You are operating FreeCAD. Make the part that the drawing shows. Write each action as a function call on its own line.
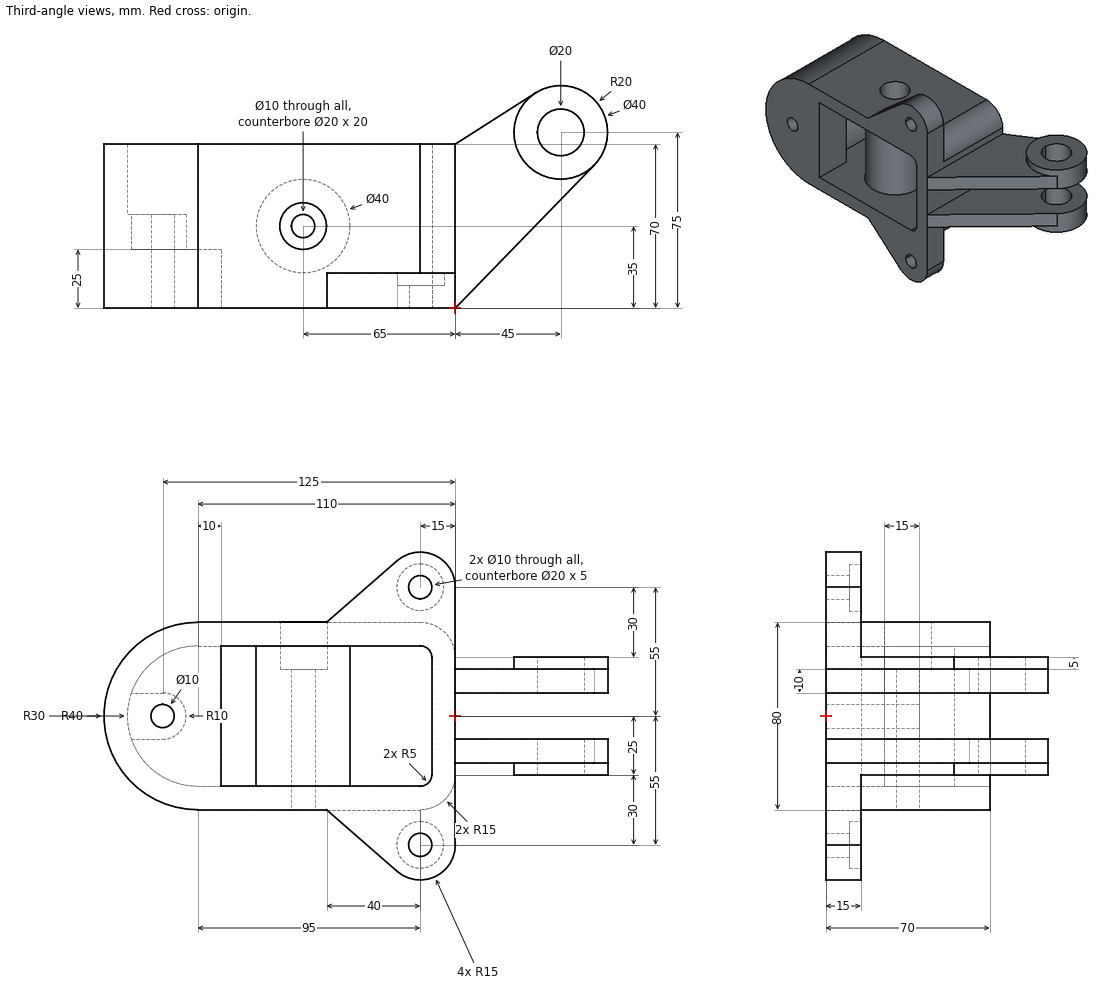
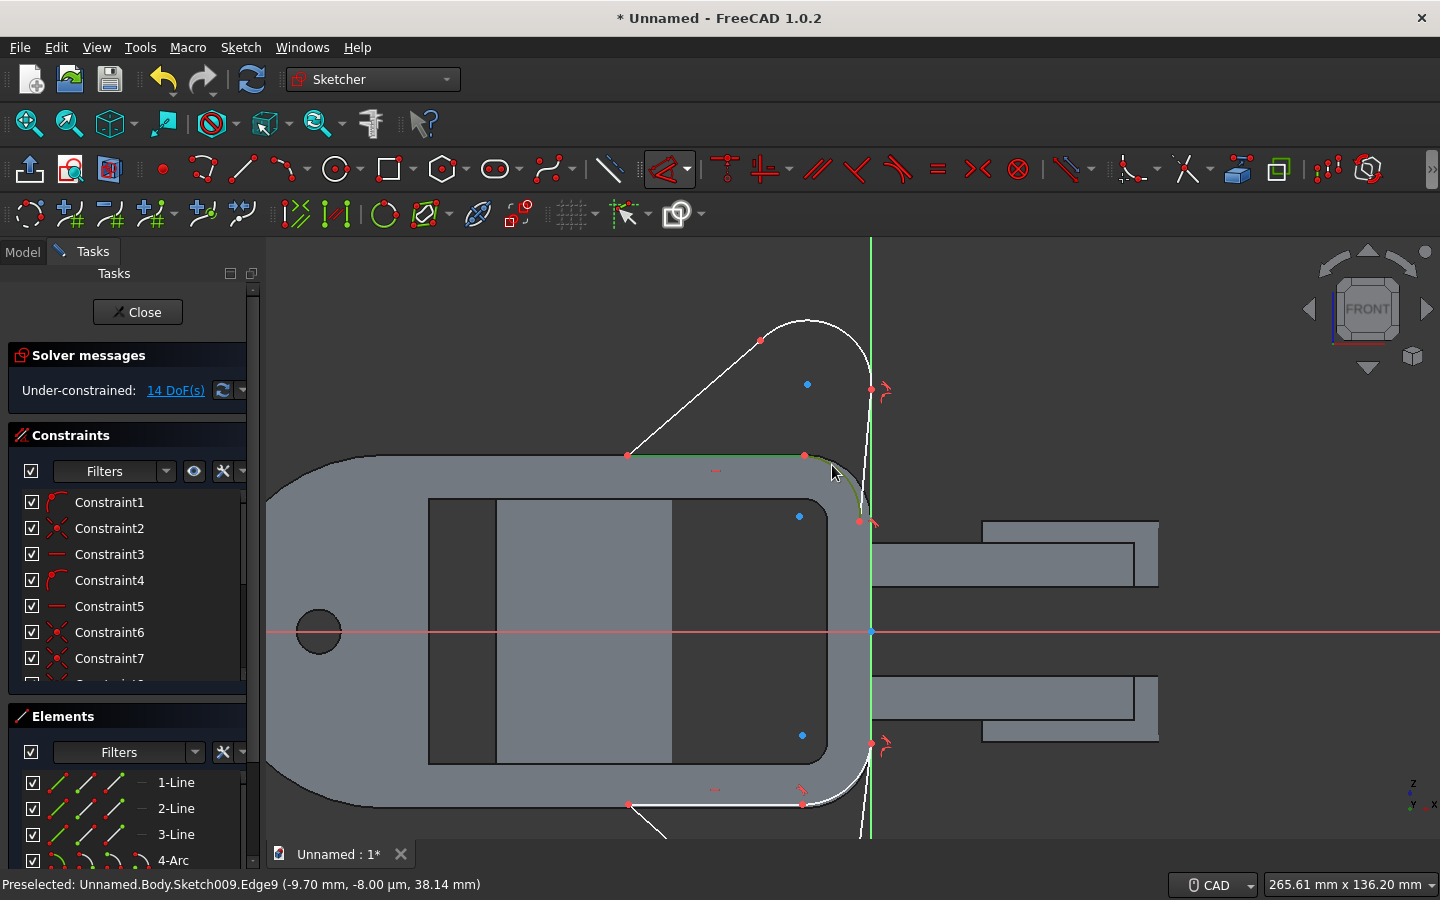
key(t)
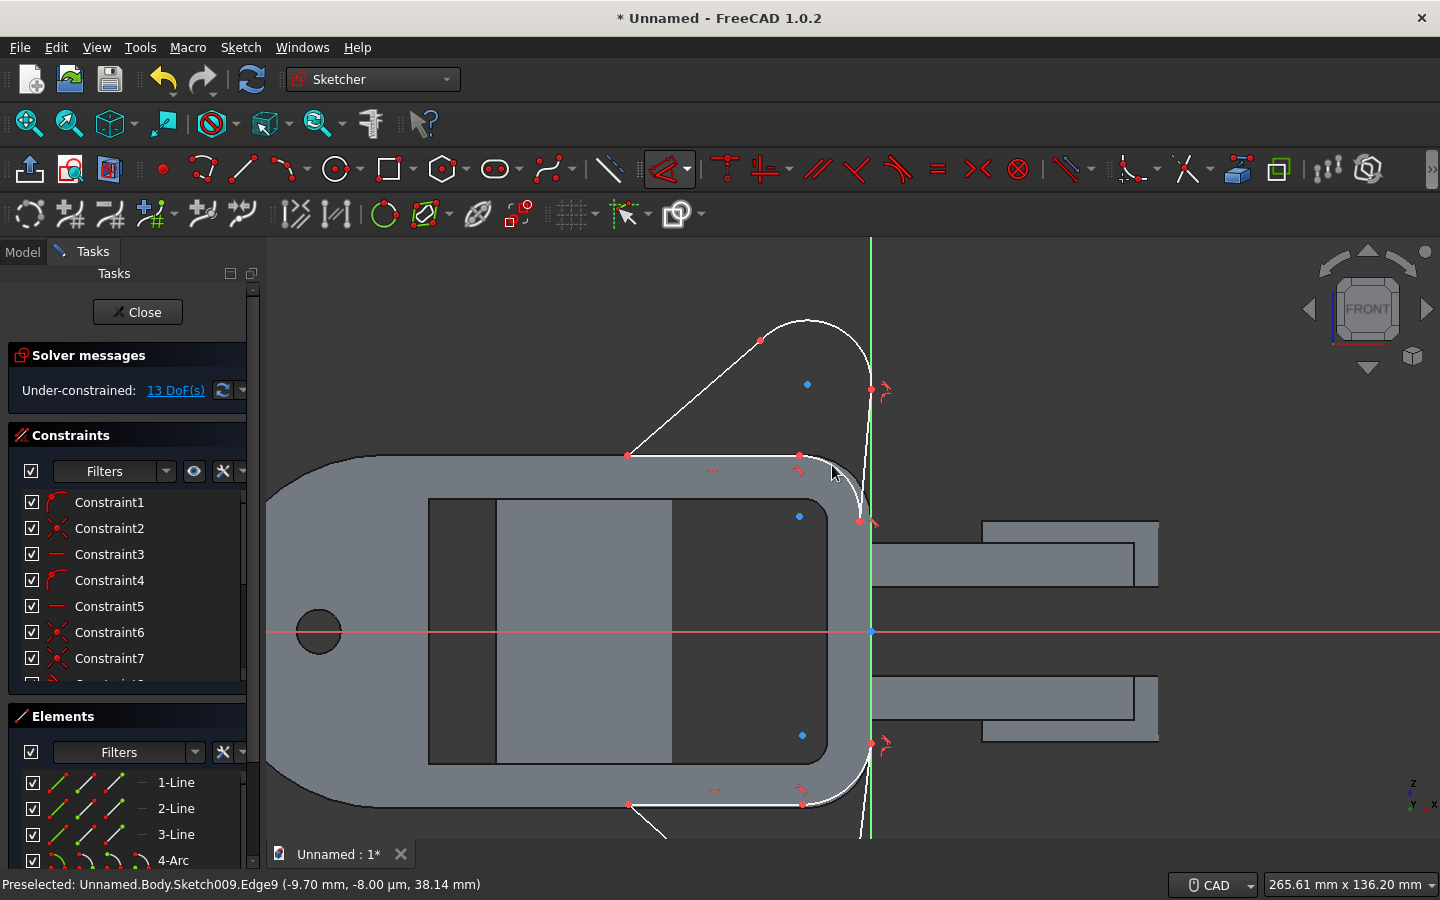
click(668, 421)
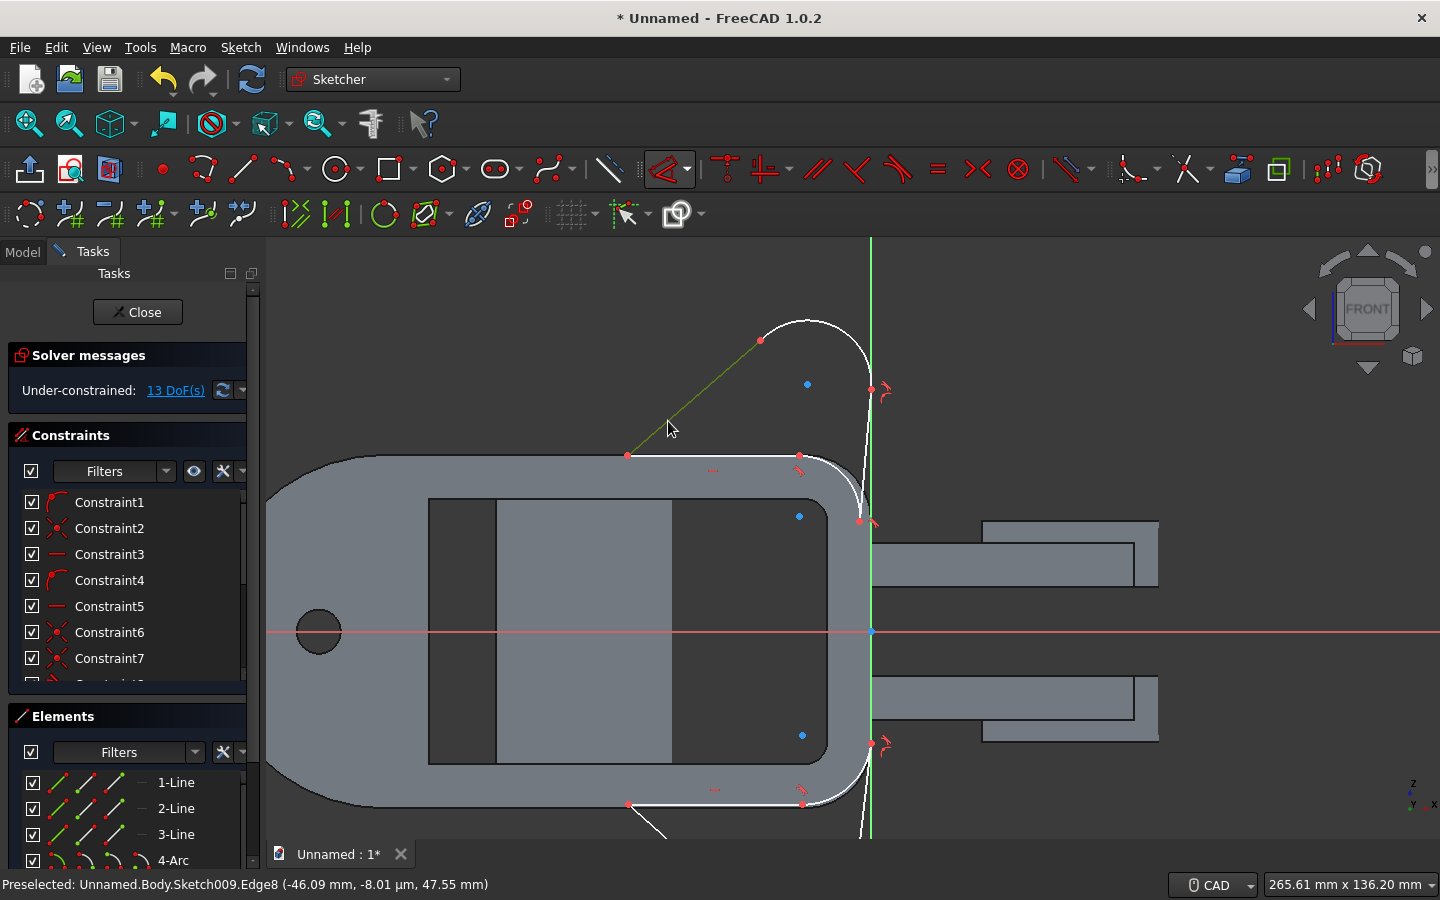
click(858, 345)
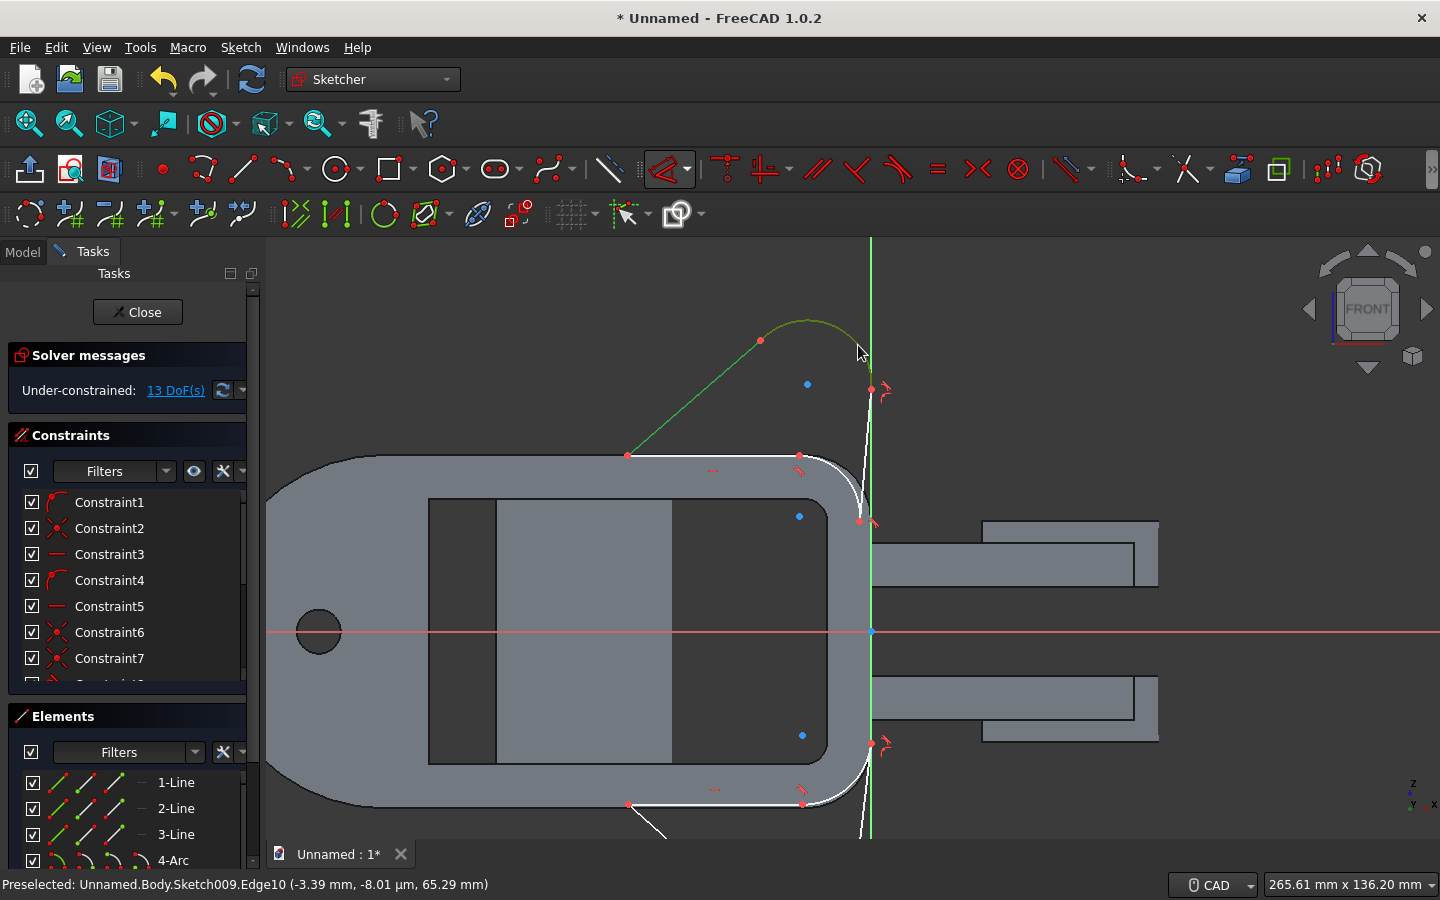
click(898, 170)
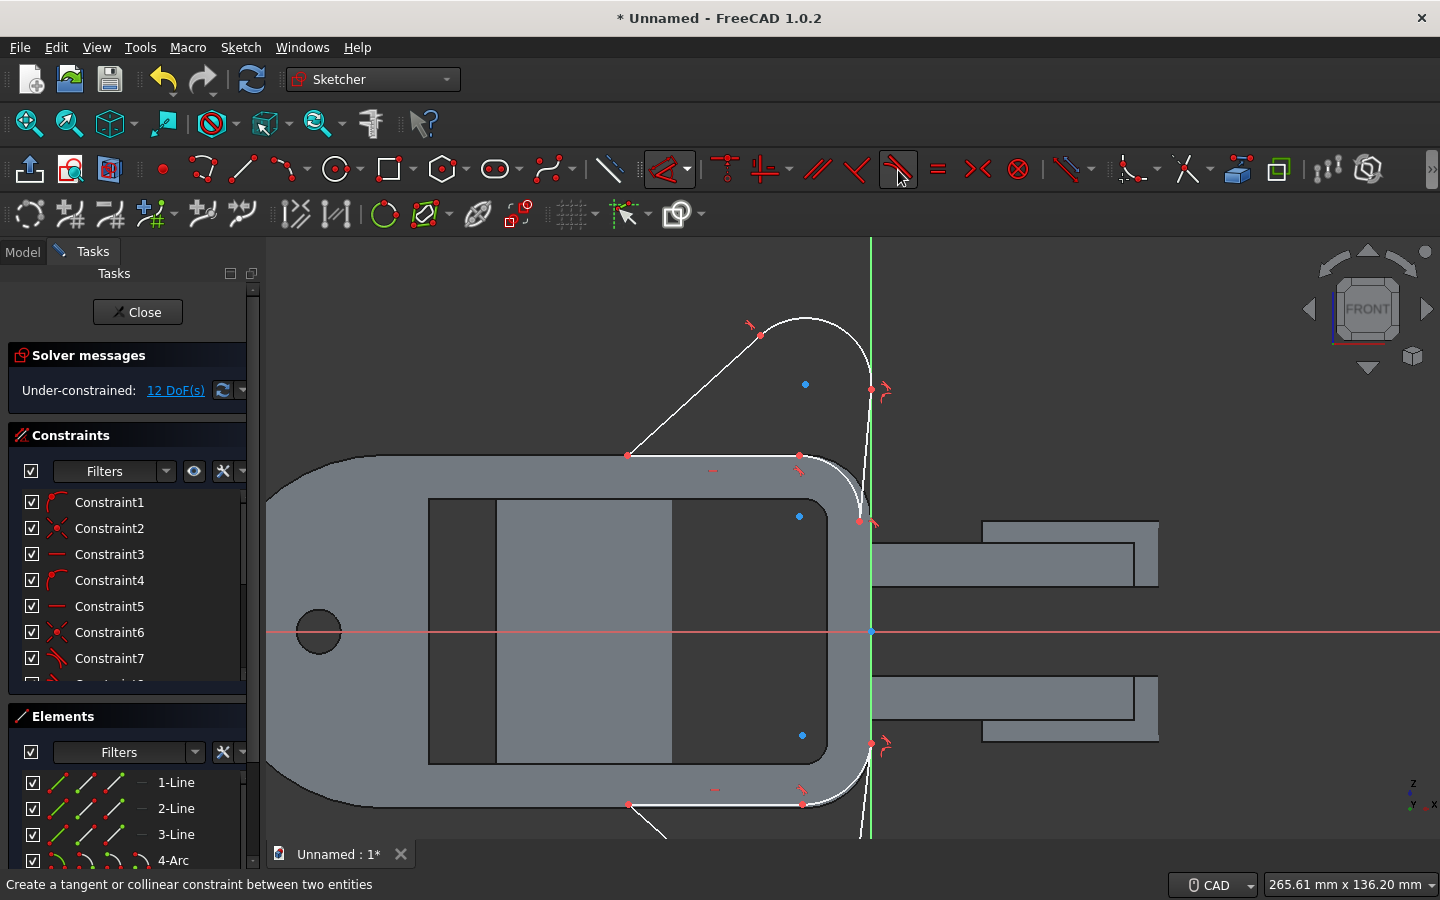
scroll(855, 348, down, 2)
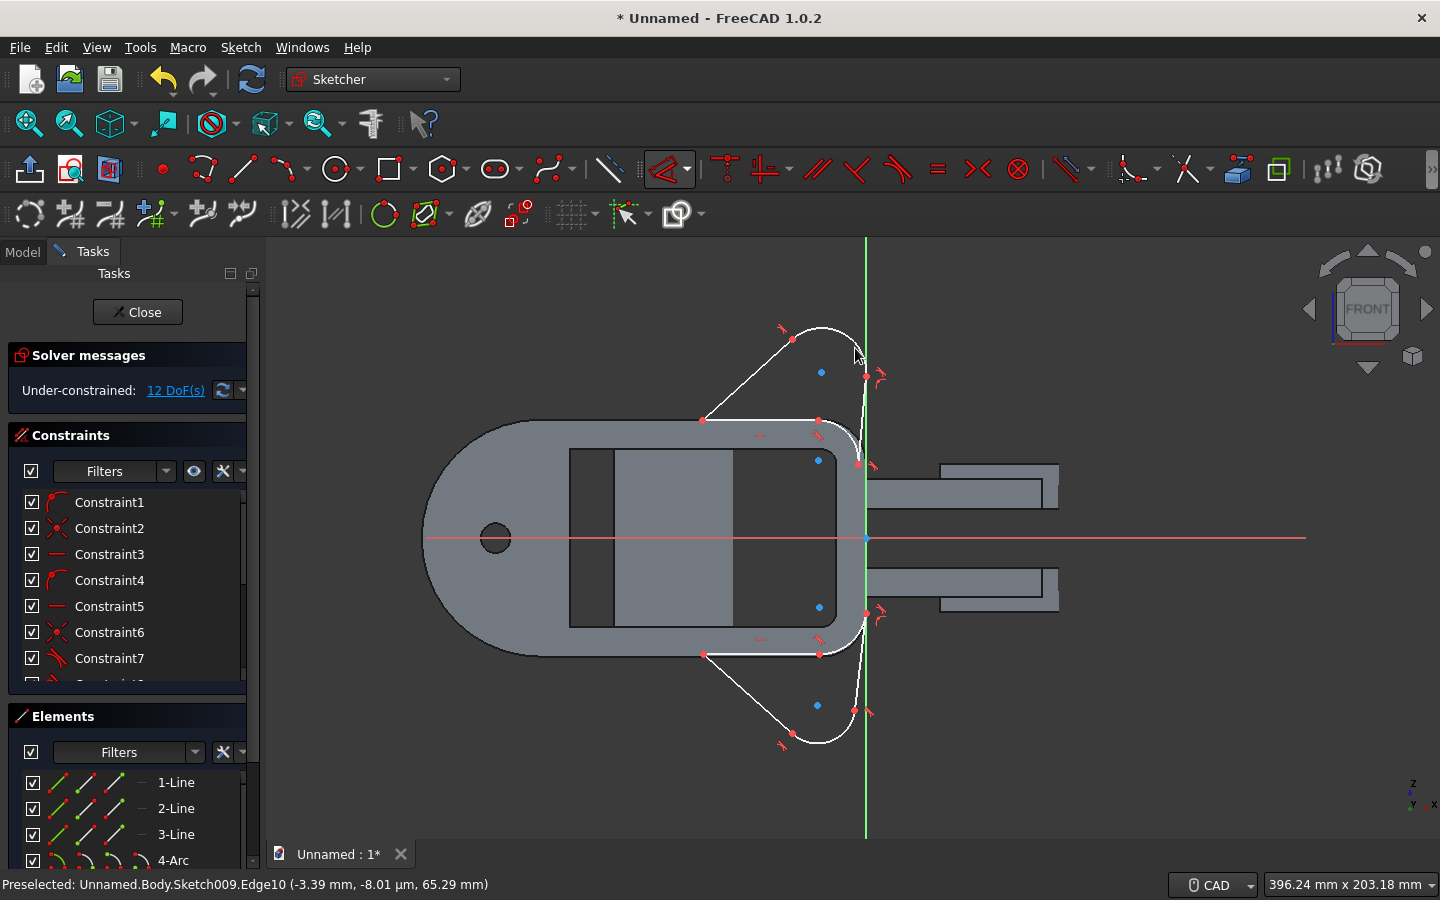
scroll(858, 681, up, 3)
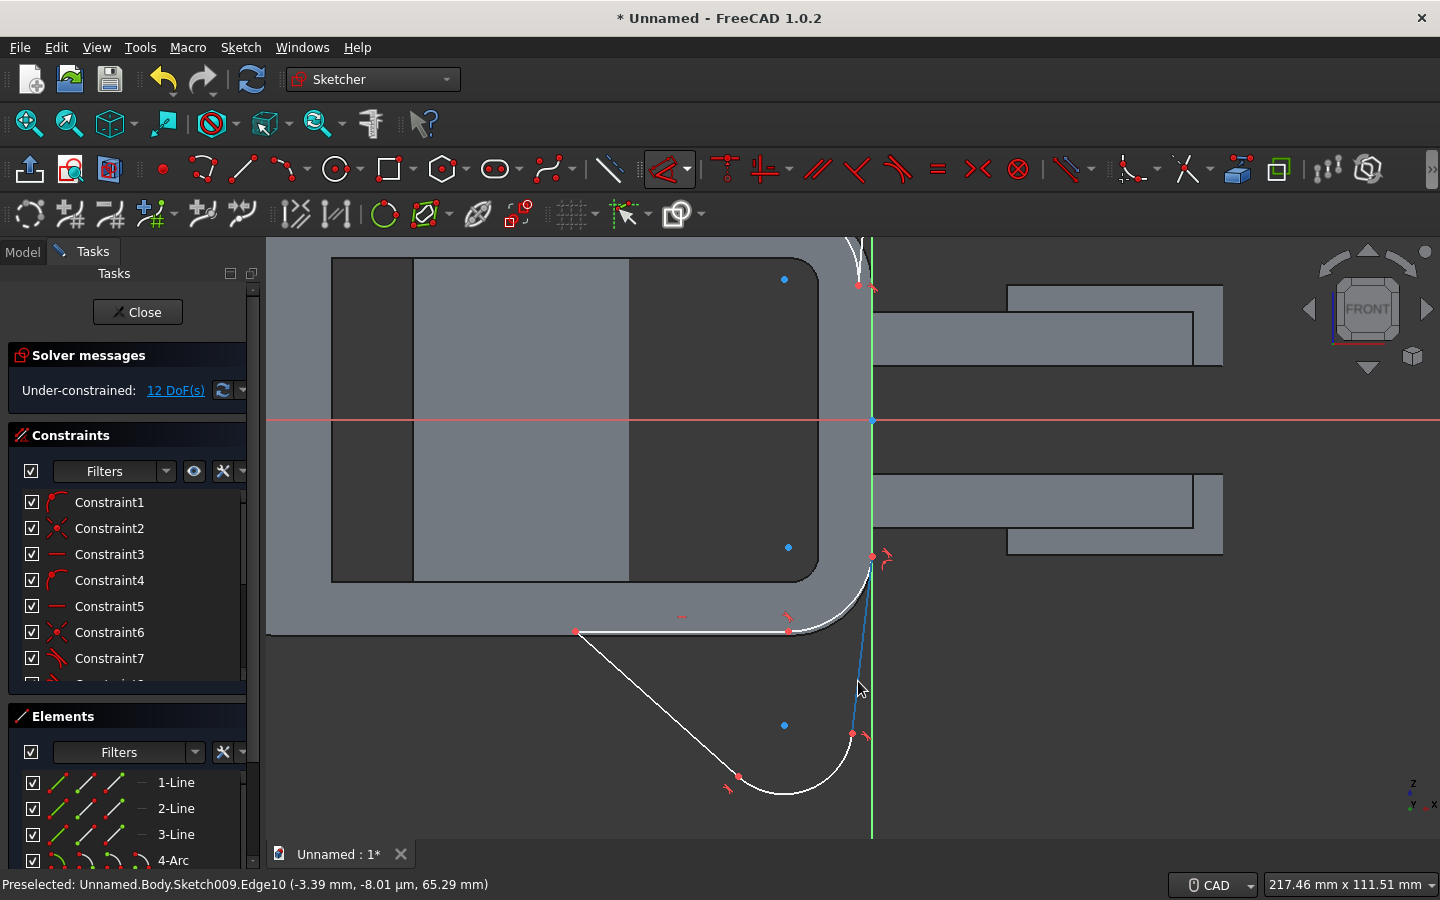
click(858, 681)